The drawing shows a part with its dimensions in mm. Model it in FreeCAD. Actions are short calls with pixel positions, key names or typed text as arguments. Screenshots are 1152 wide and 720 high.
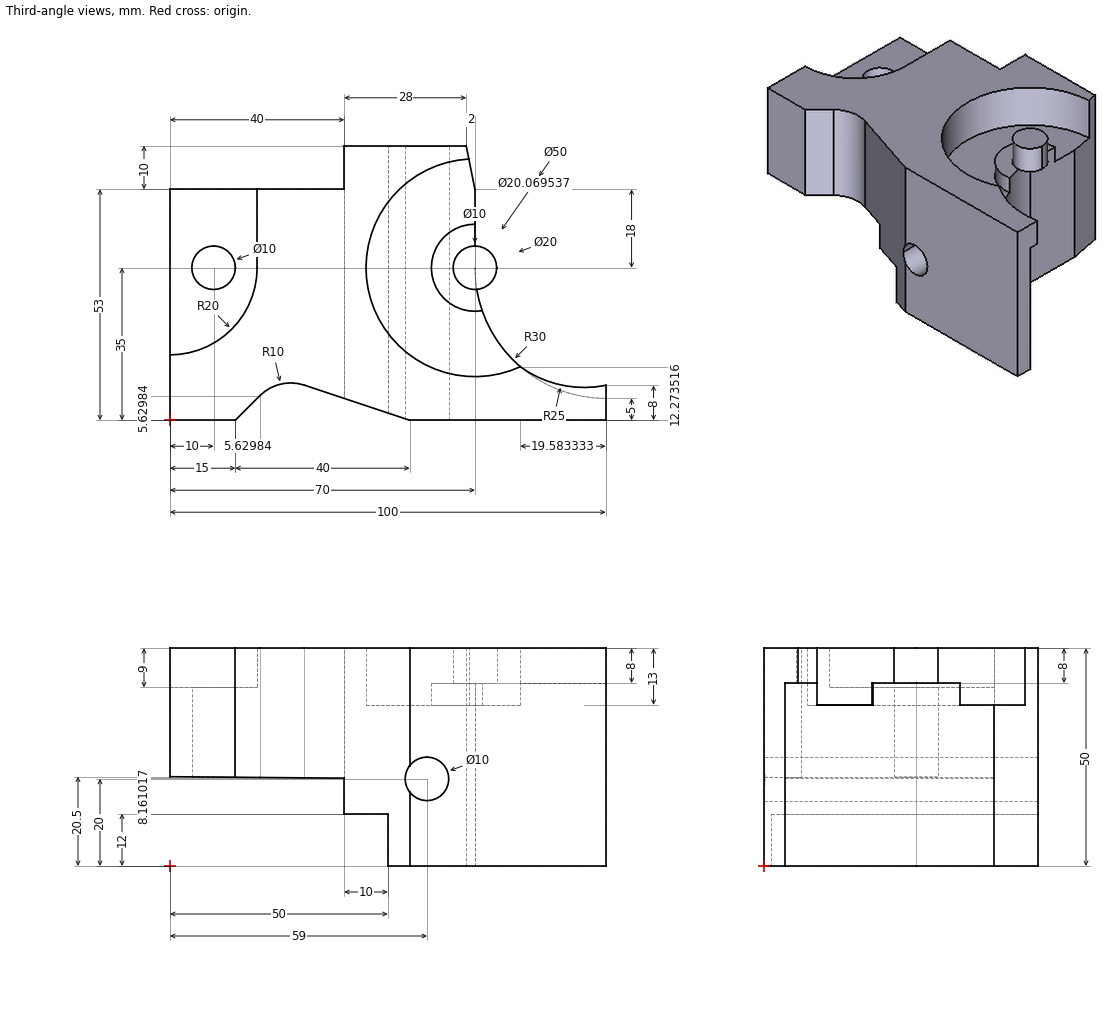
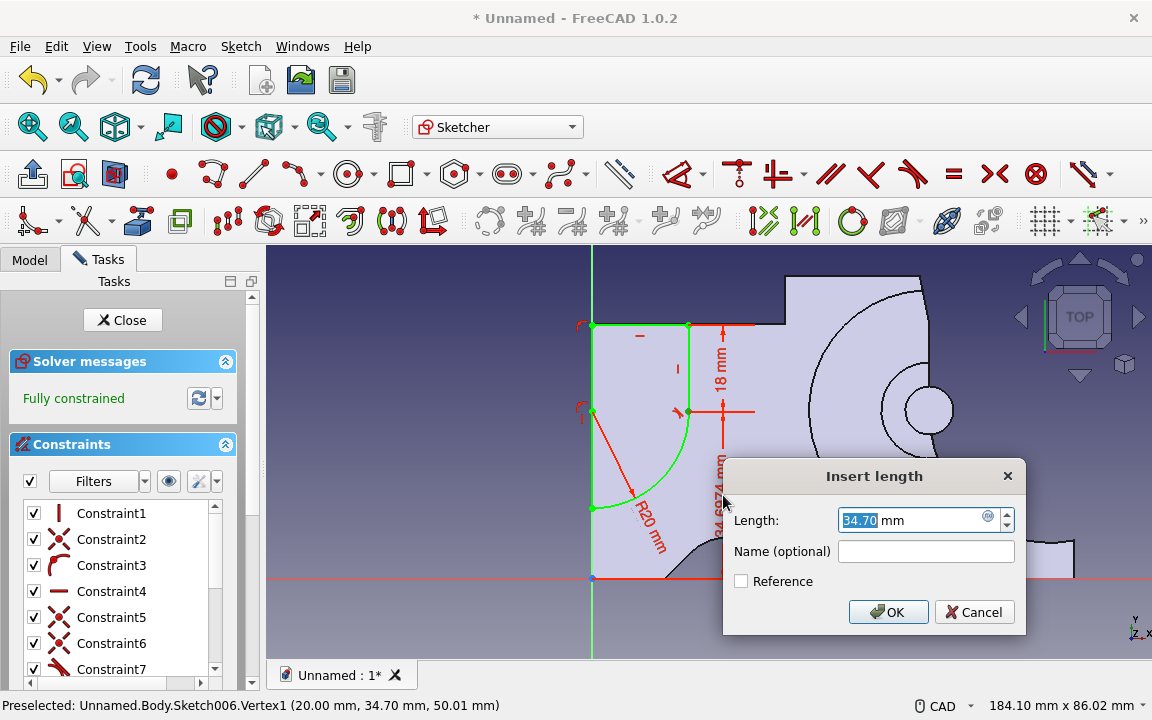
text(35)
key(Return)
key(Escape)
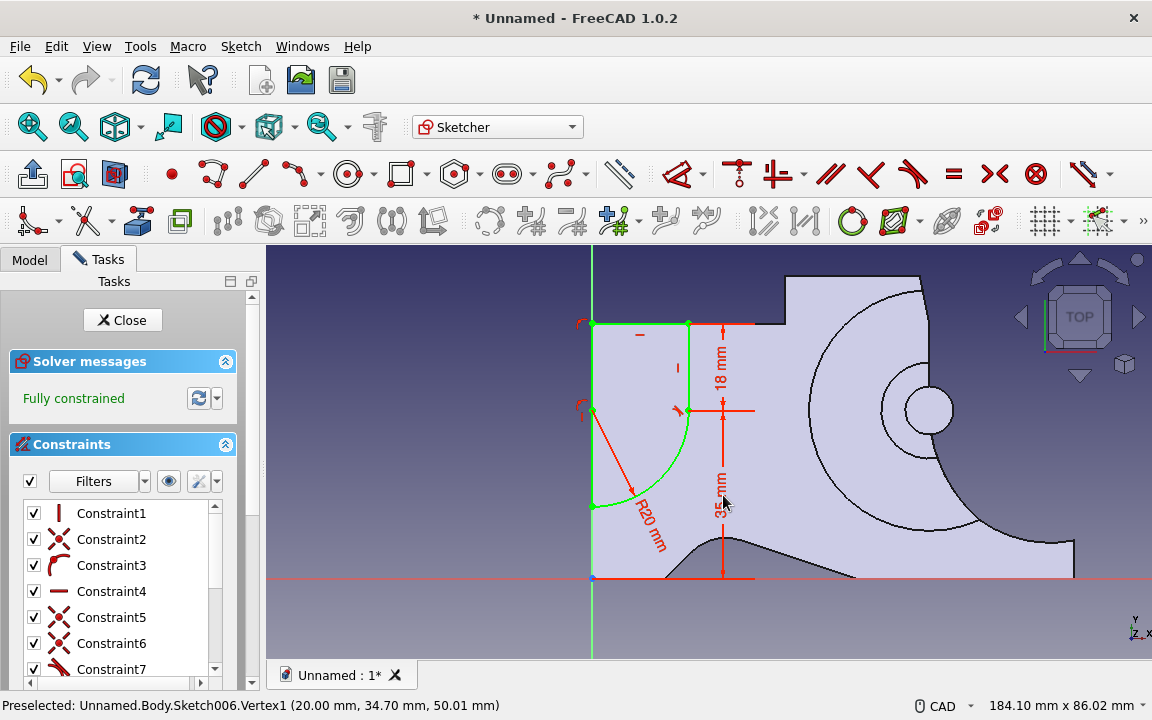
click(123, 320)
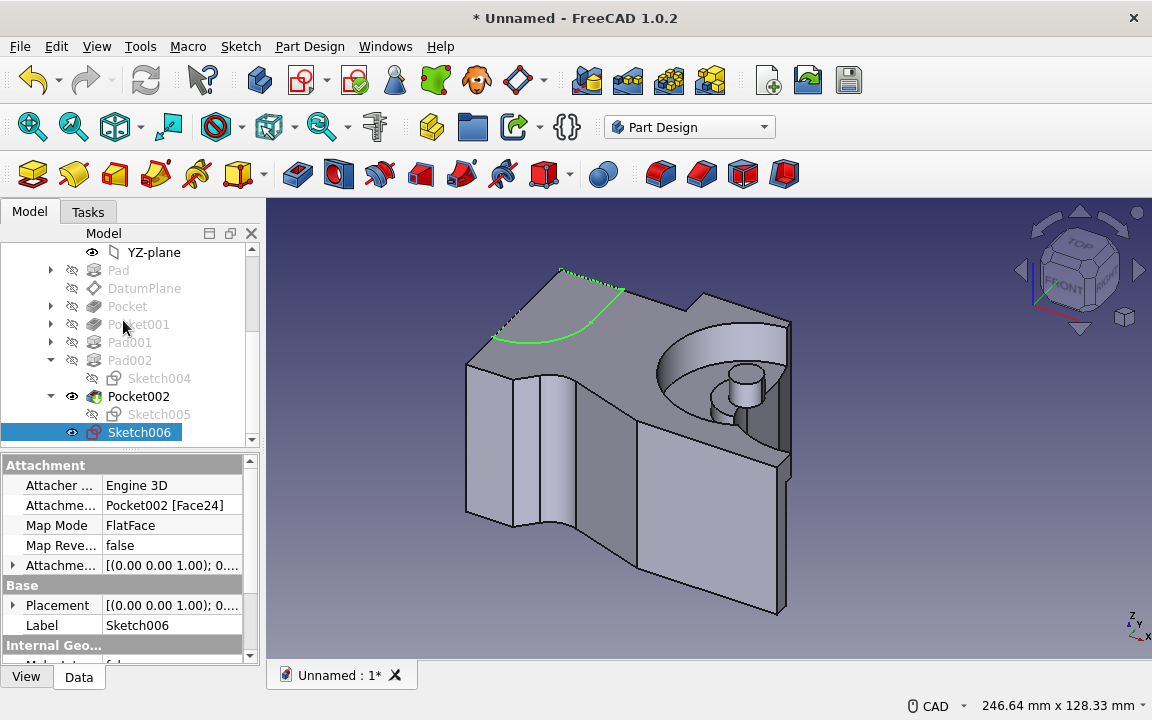
click(298, 174)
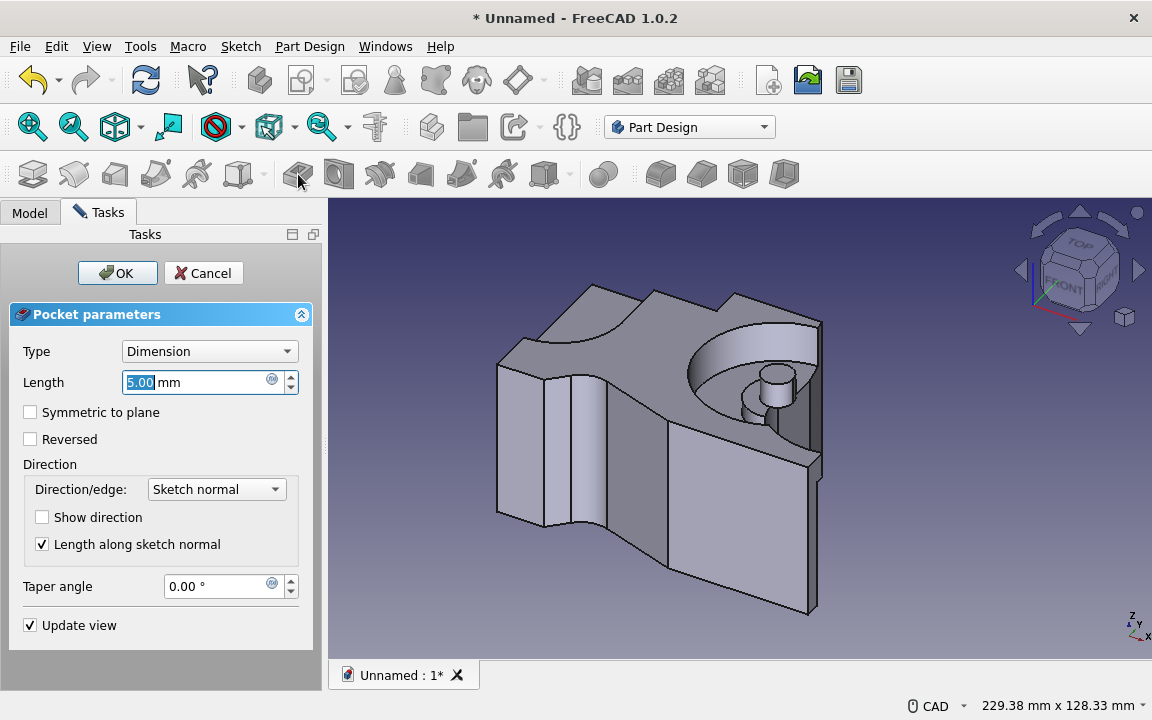
text(9)
key(Tab)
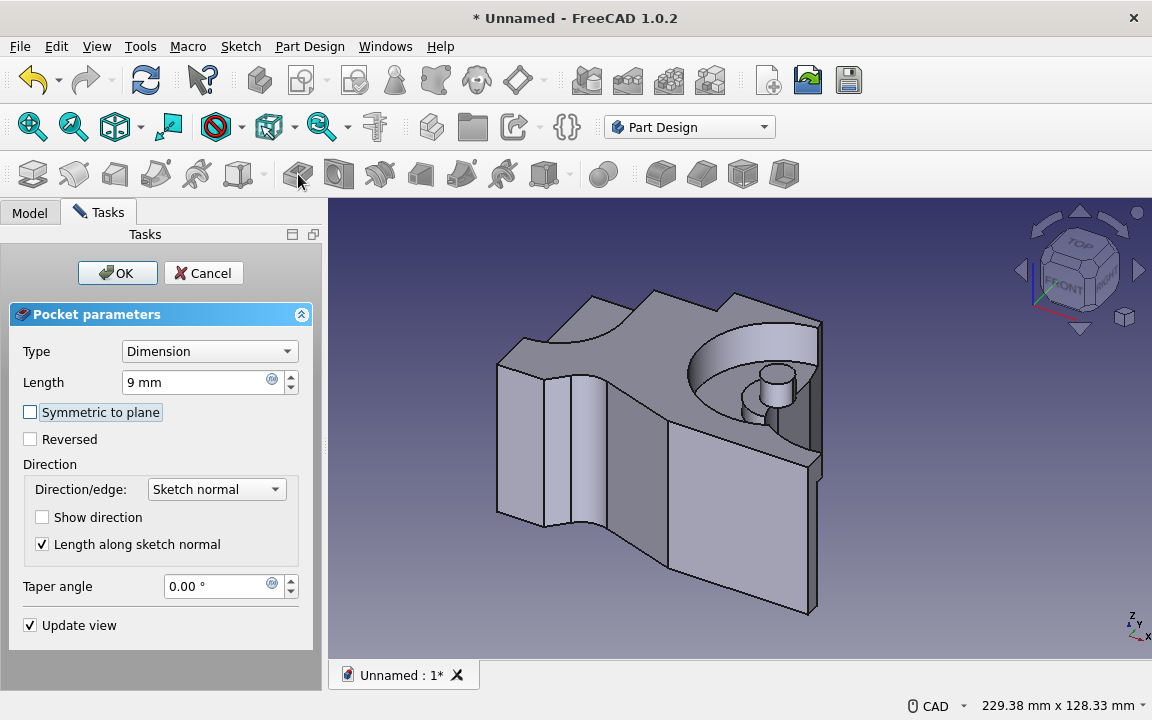
click(118, 273)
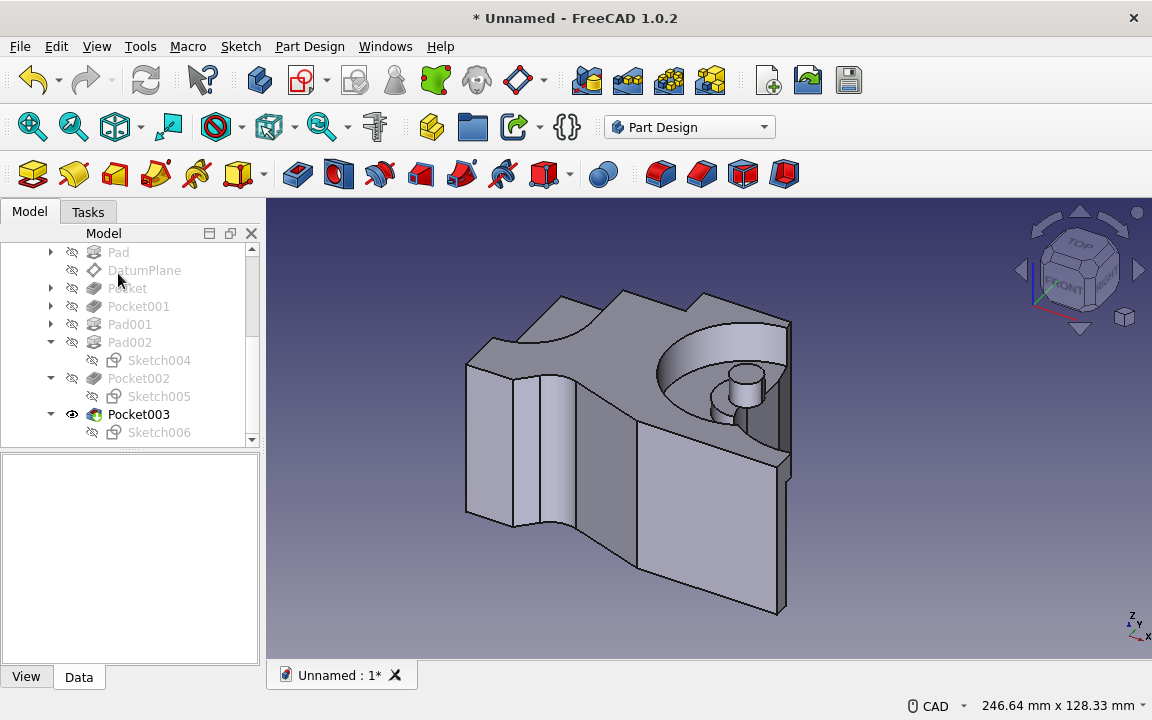
click(578, 320)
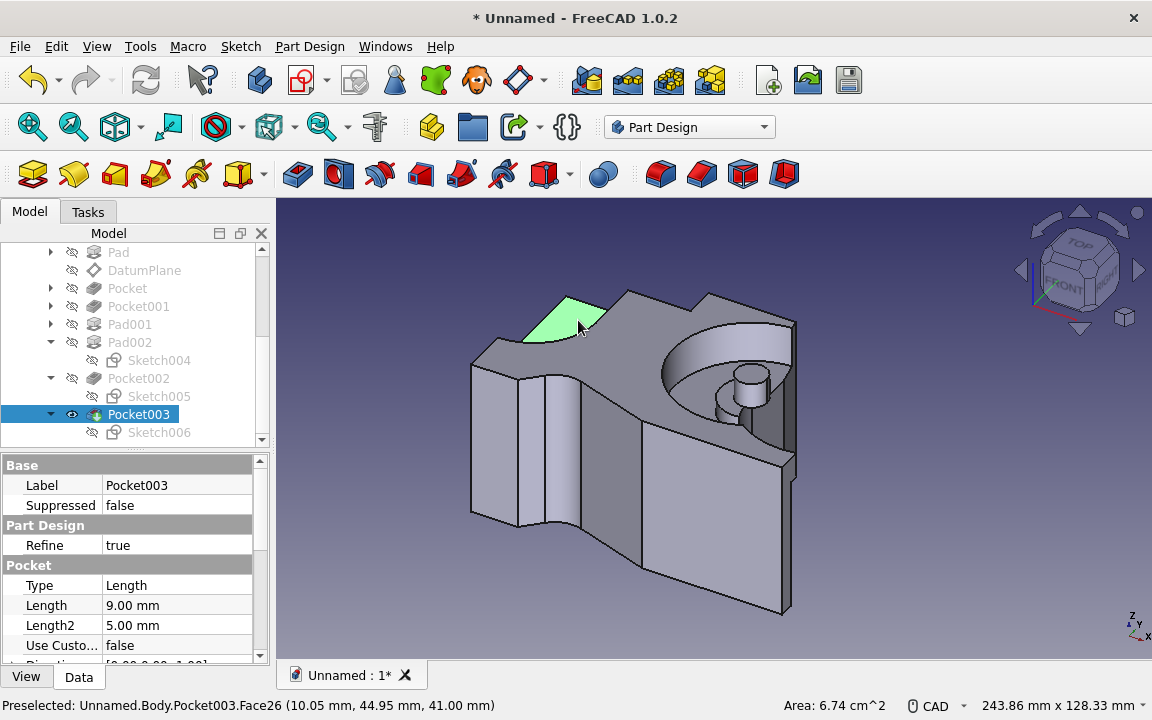
click(300, 80)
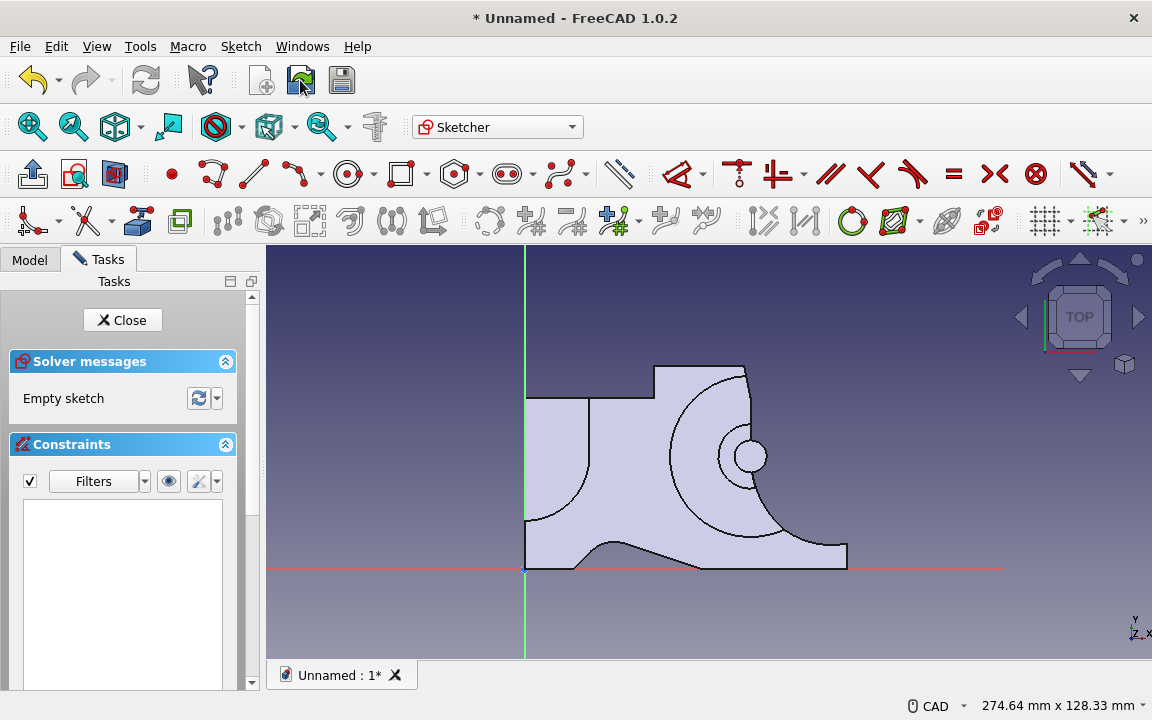
key(q)
key(s)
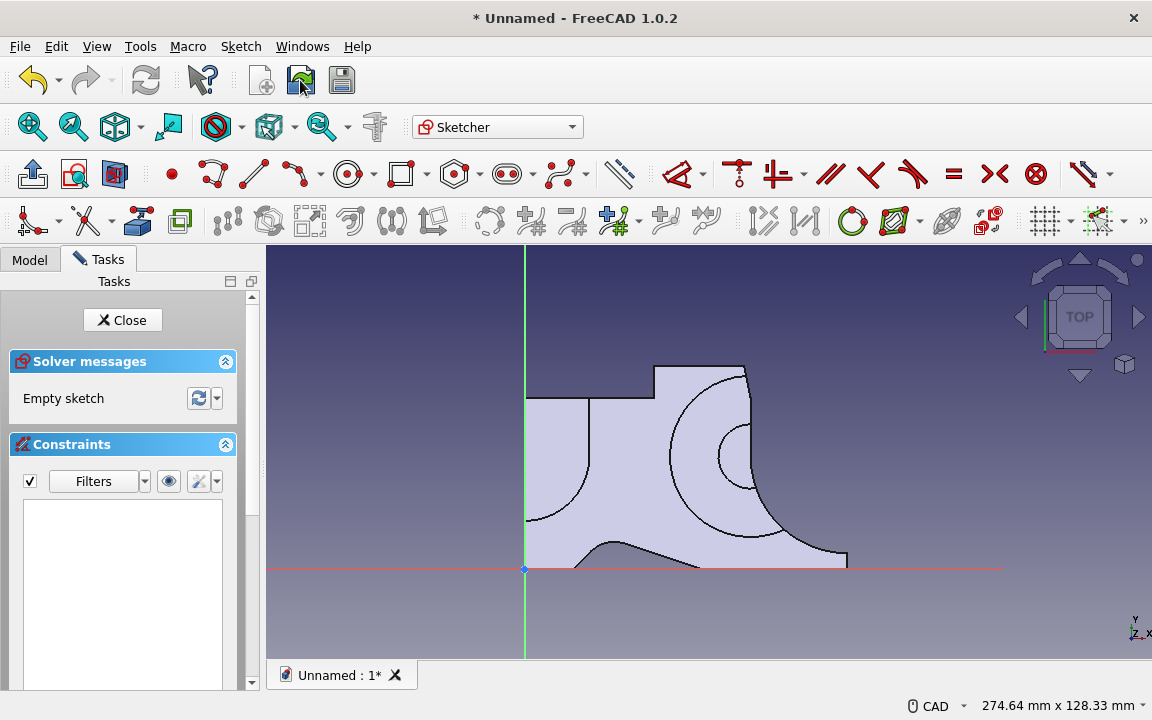
scroll(544, 457, up, 10)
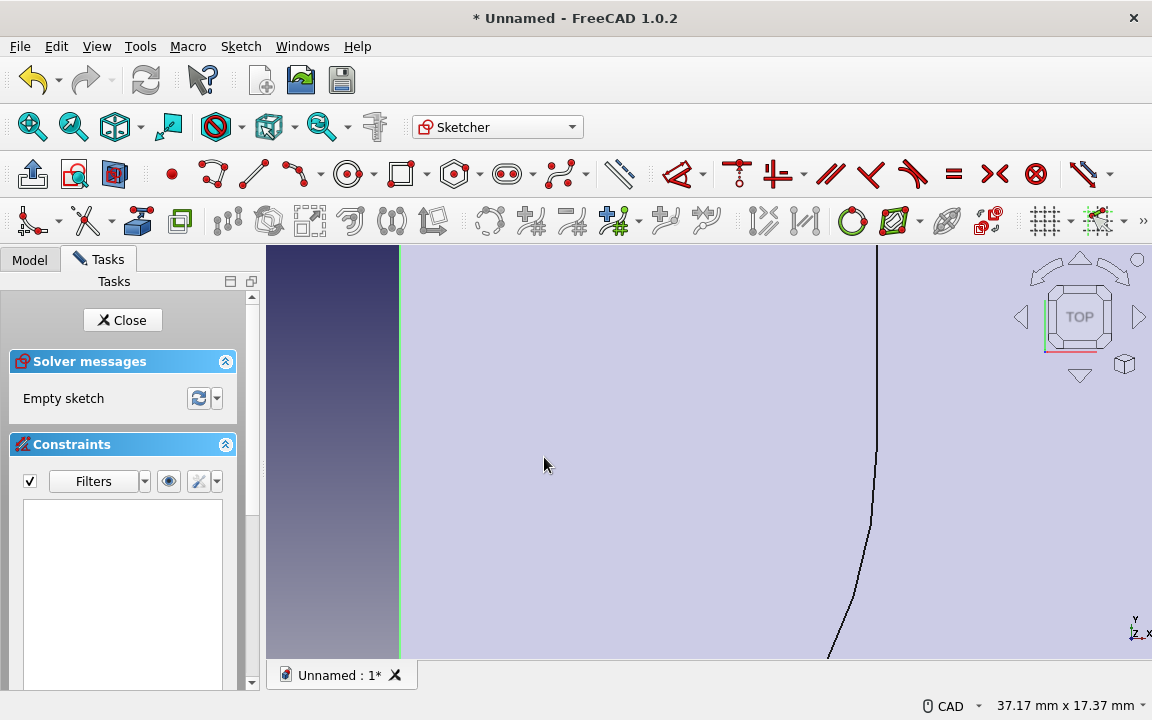
key(g)
key(c)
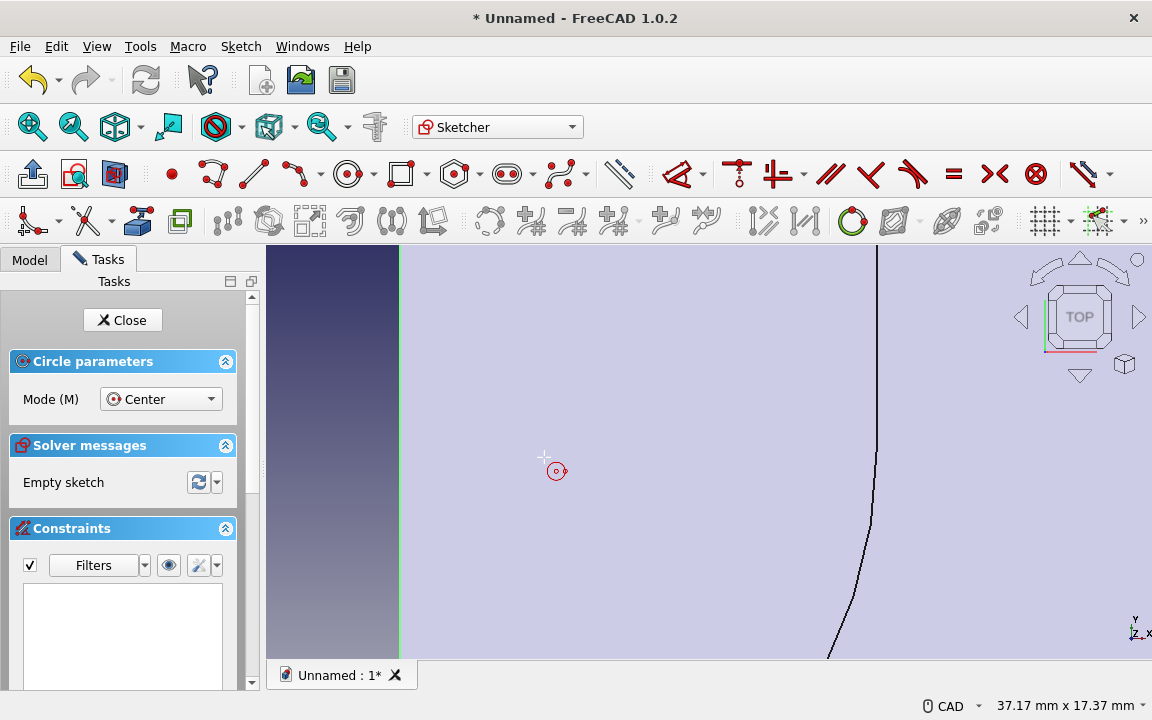
click(638, 450)
click(723, 365)
key(Escape)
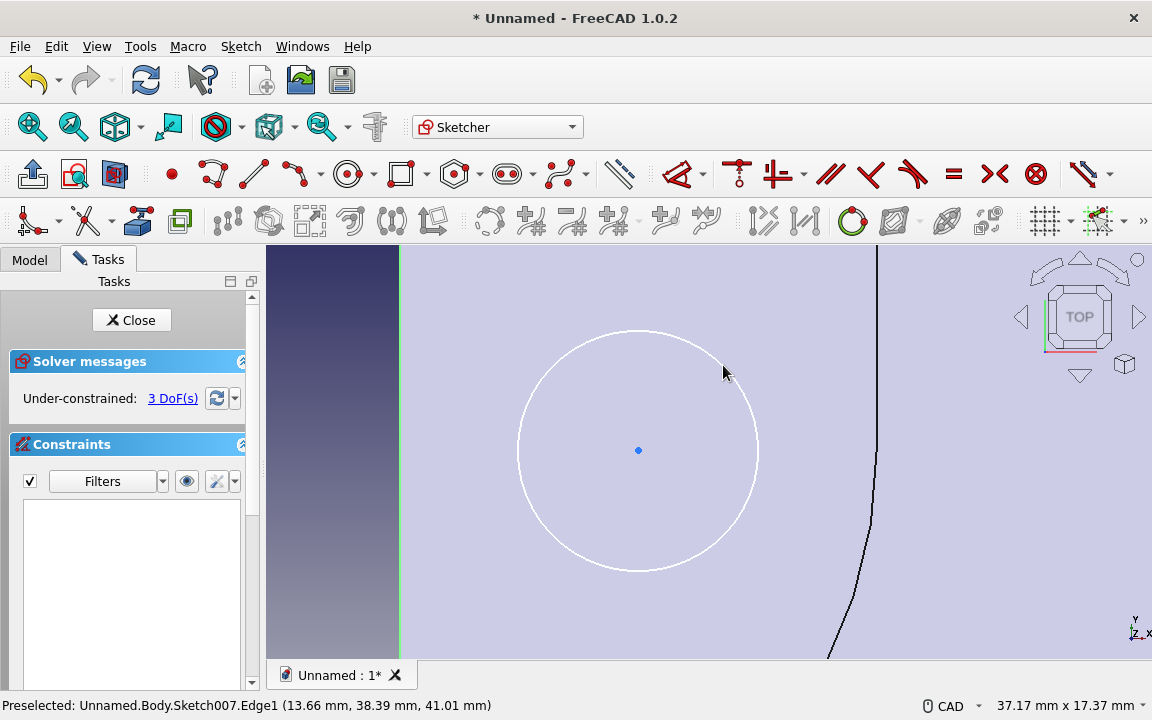
key(d)